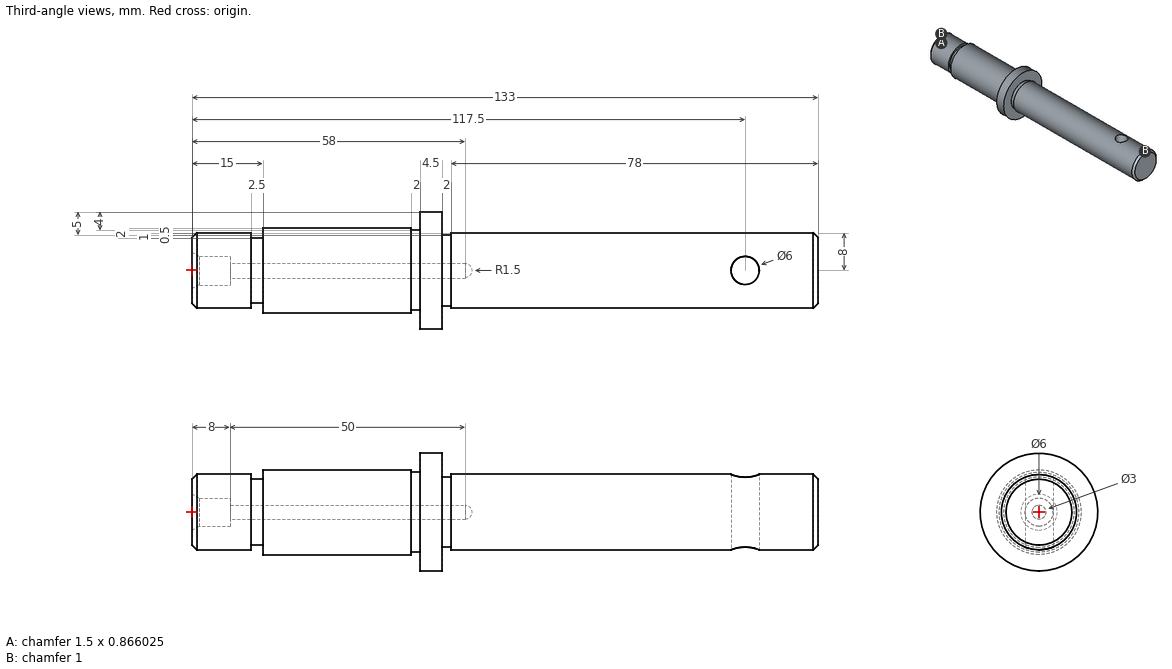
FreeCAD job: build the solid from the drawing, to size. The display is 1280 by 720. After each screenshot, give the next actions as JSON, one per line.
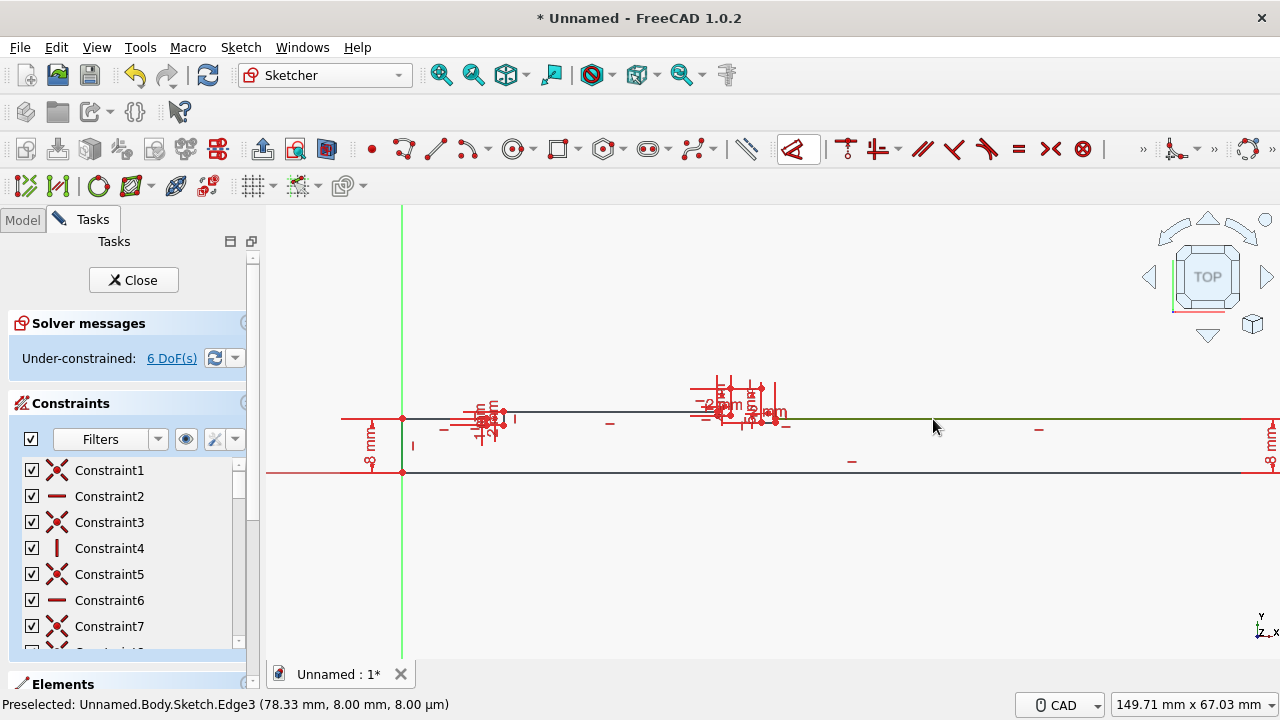
{"action": "left_click", "coordinate": [814, 150]}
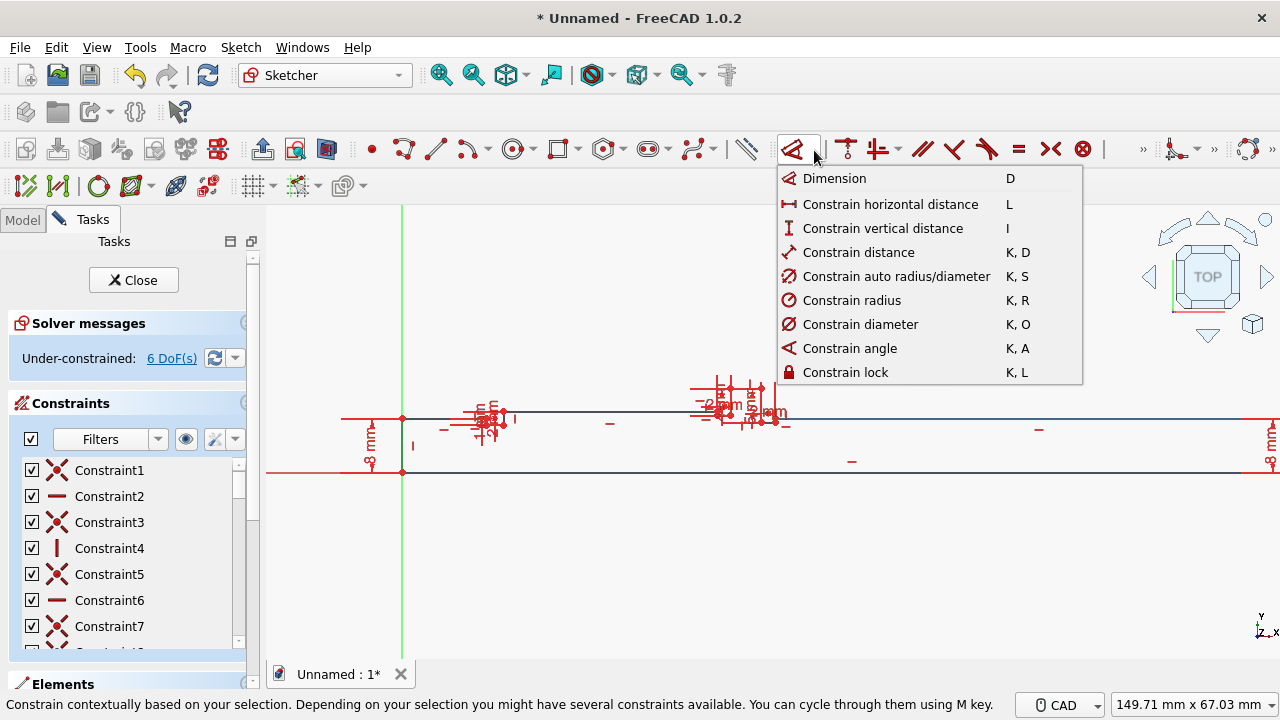
{"action": "left_click", "coordinate": [930, 204]}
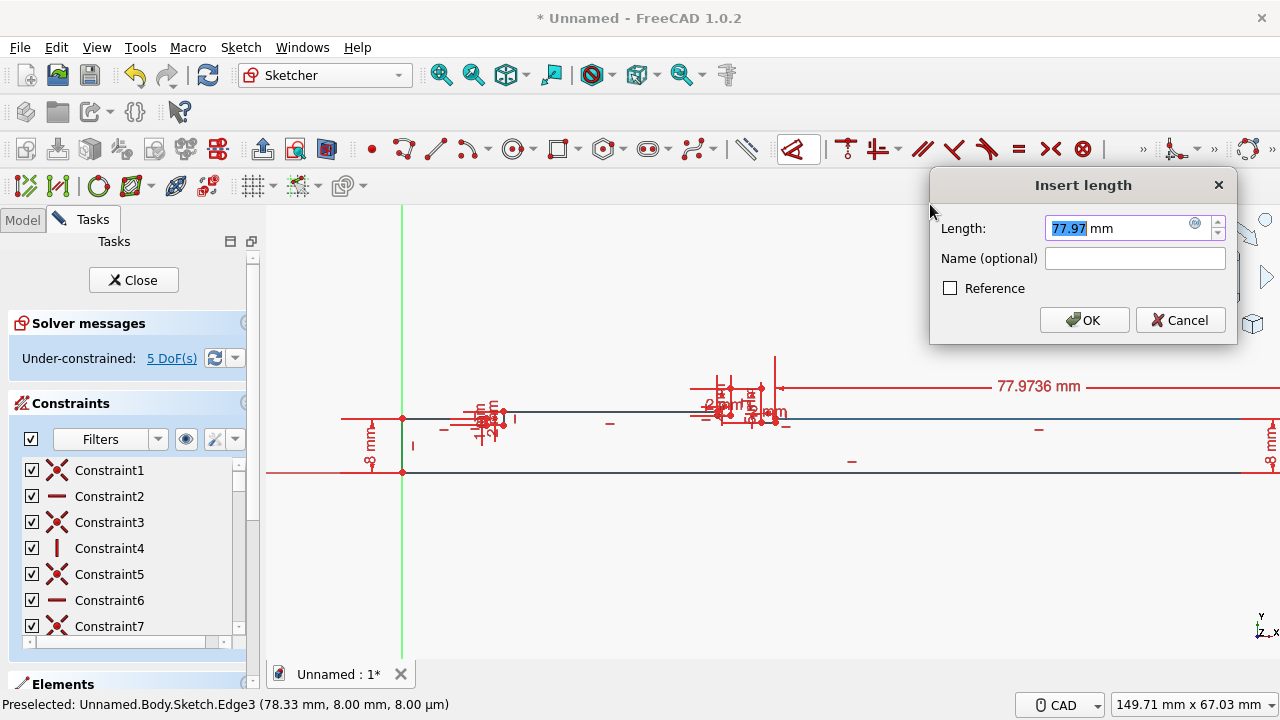
{"action": "type", "text": "78"}
{"action": "key", "text": "Return"}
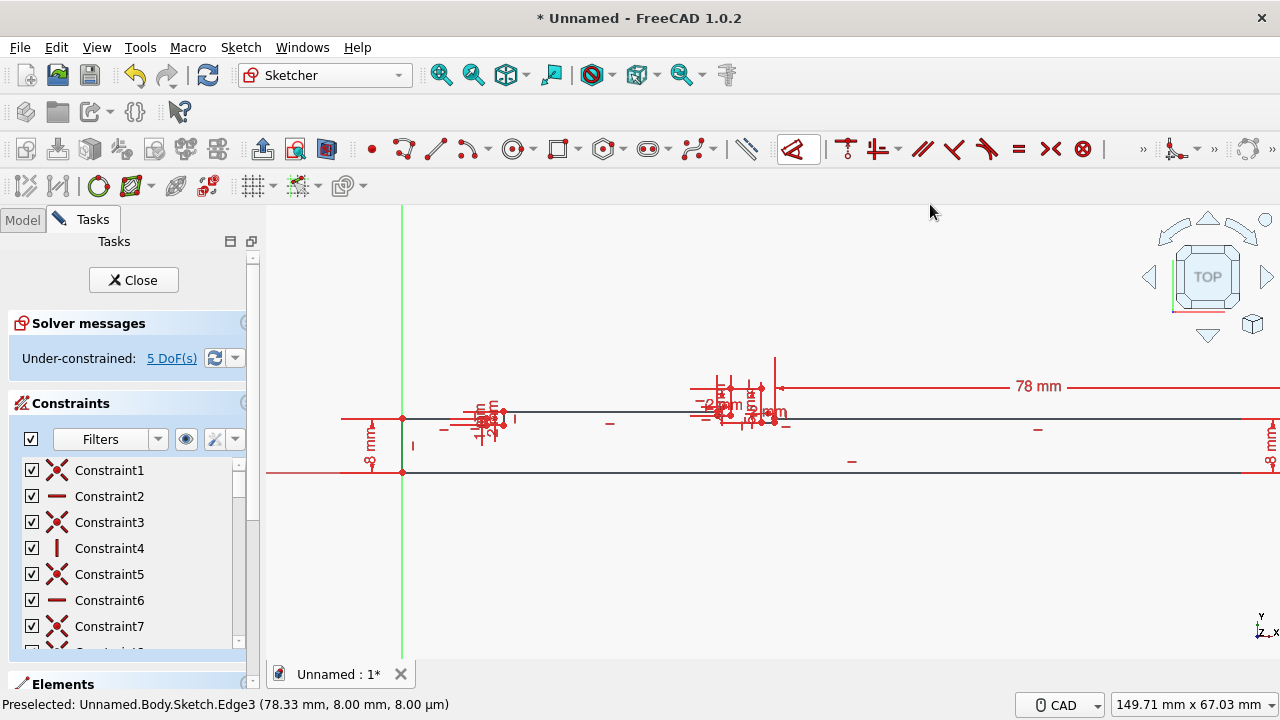
{"action": "left_click", "coordinate": [673, 473]}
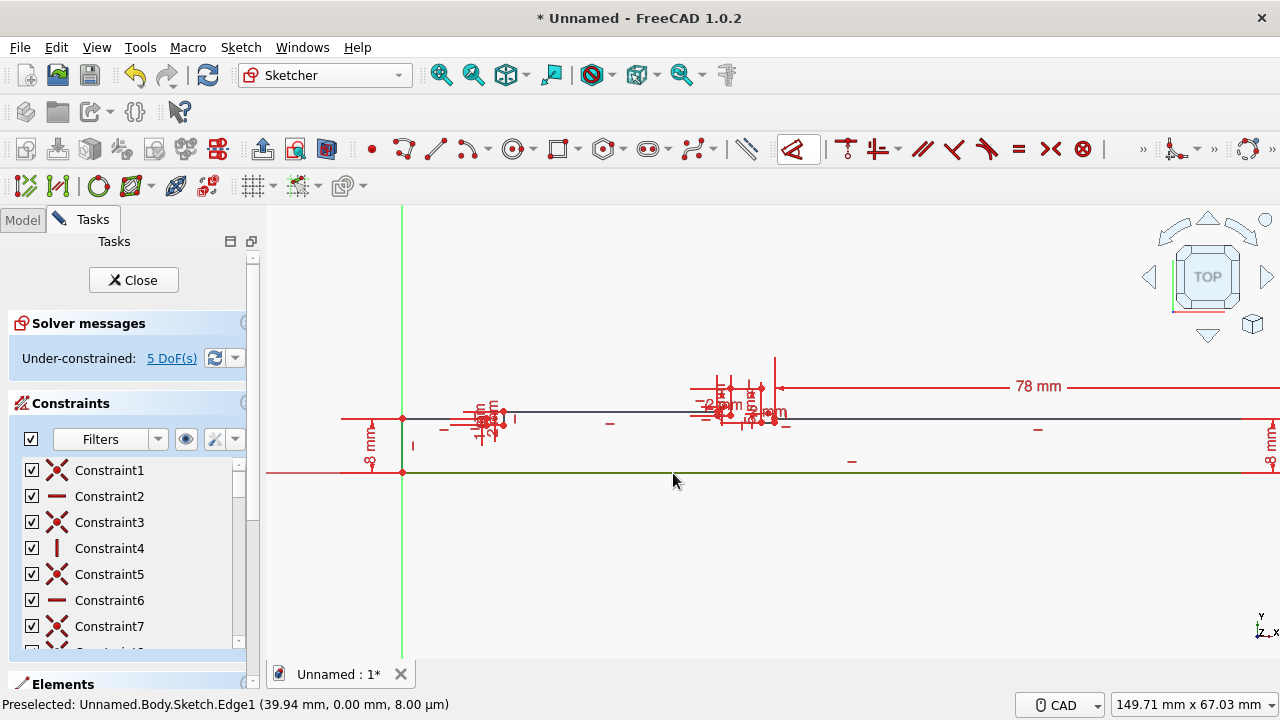
{"action": "left_click", "coordinate": [814, 150]}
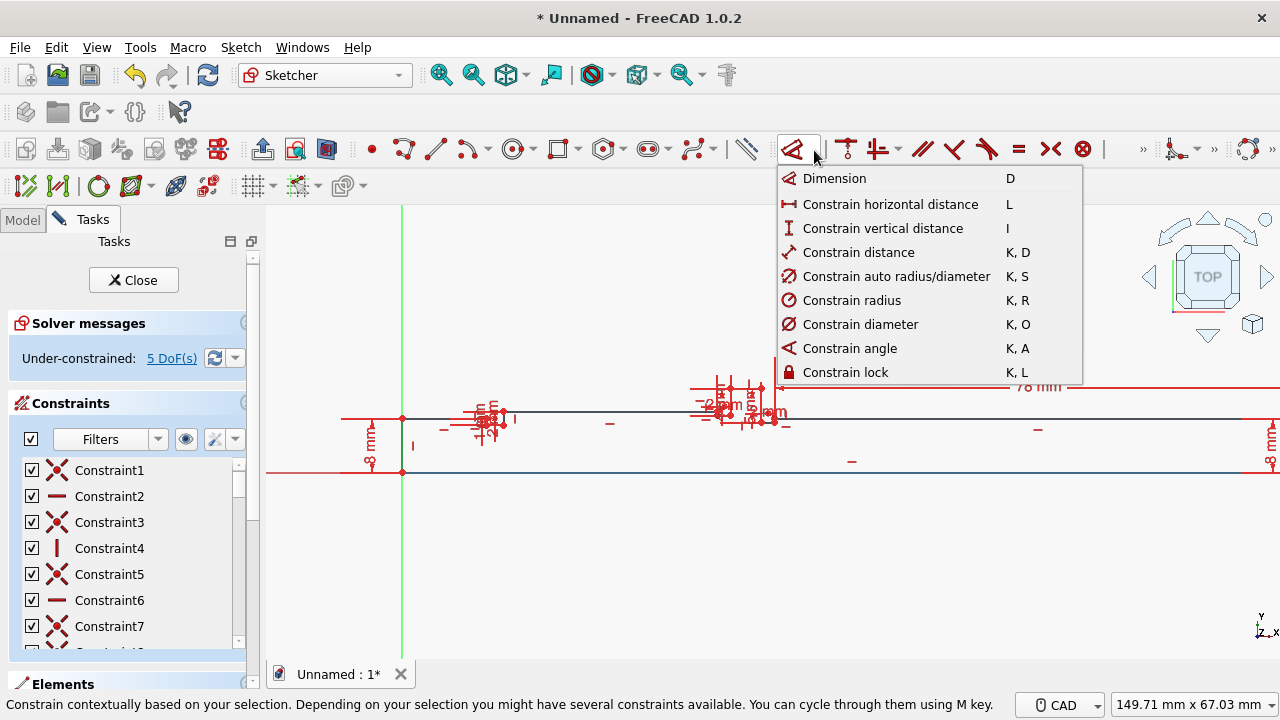
{"action": "left_click", "coordinate": [930, 204]}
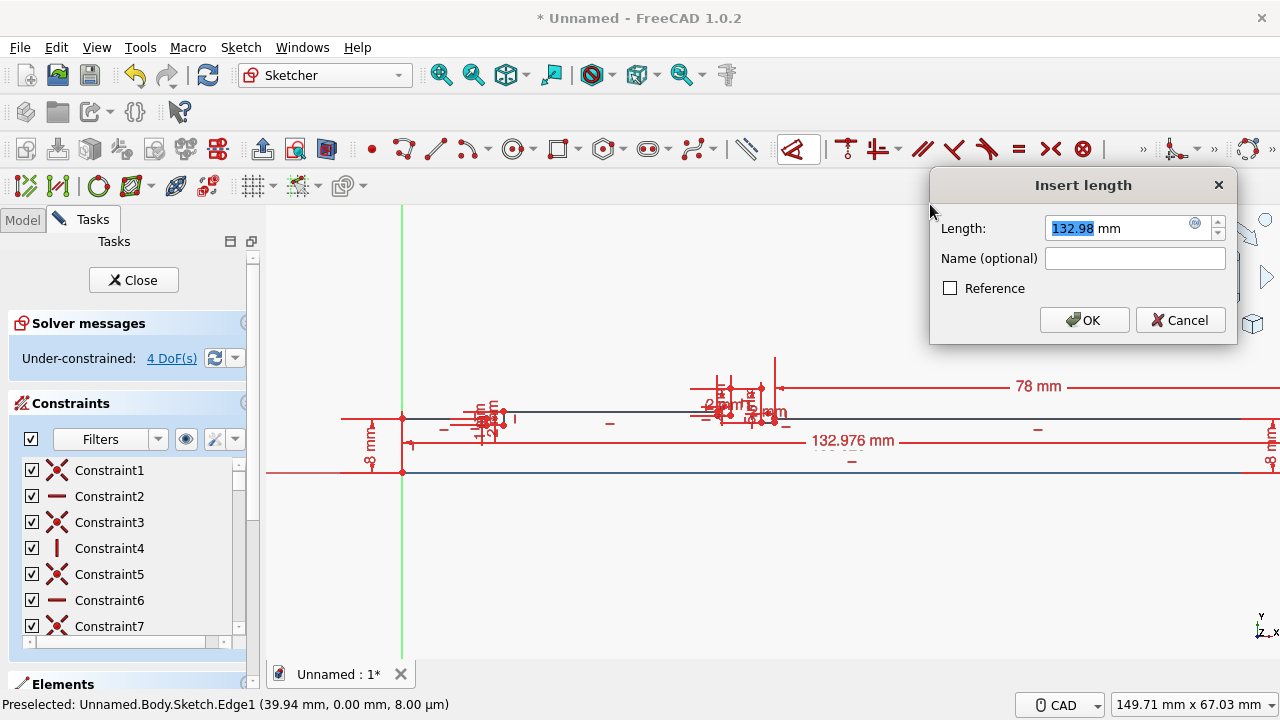
{"action": "type", "text": "133"}
{"action": "key", "text": "Return"}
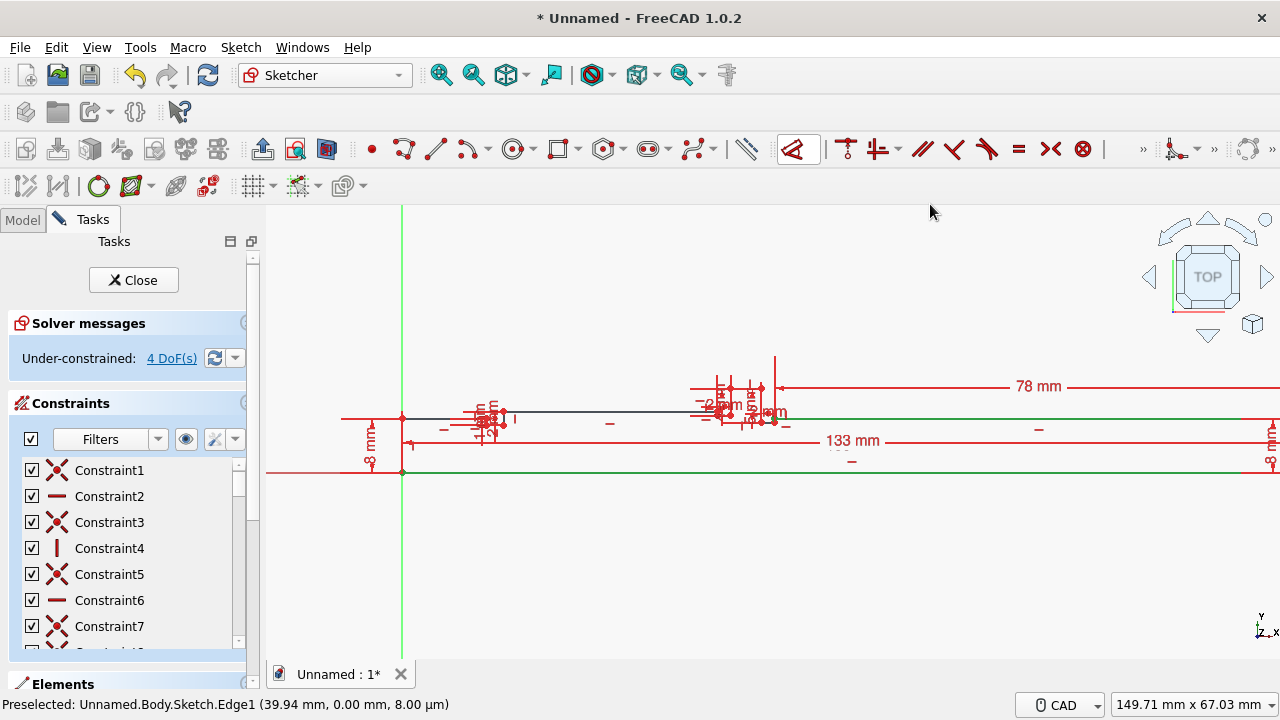
{"action": "scroll", "coordinate": [775, 421], "scroll_direction": "up", "scroll_amount": 13}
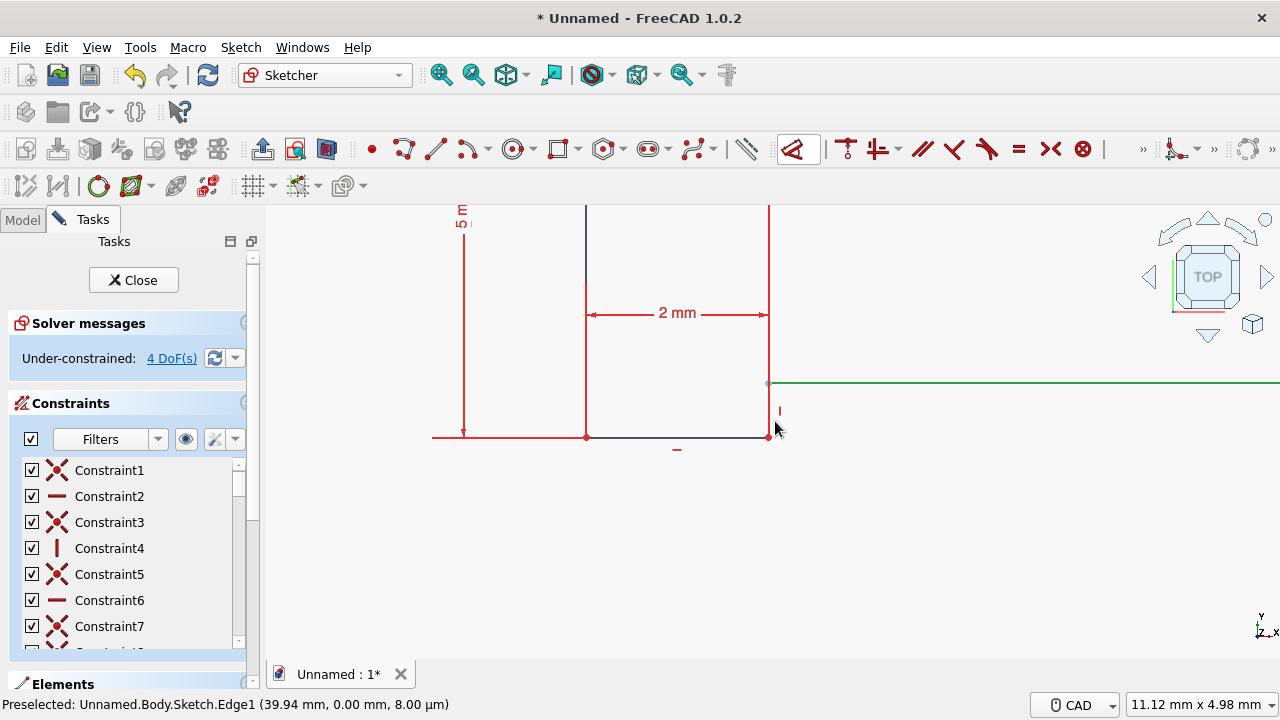
{"action": "left_click", "coordinate": [769, 411]}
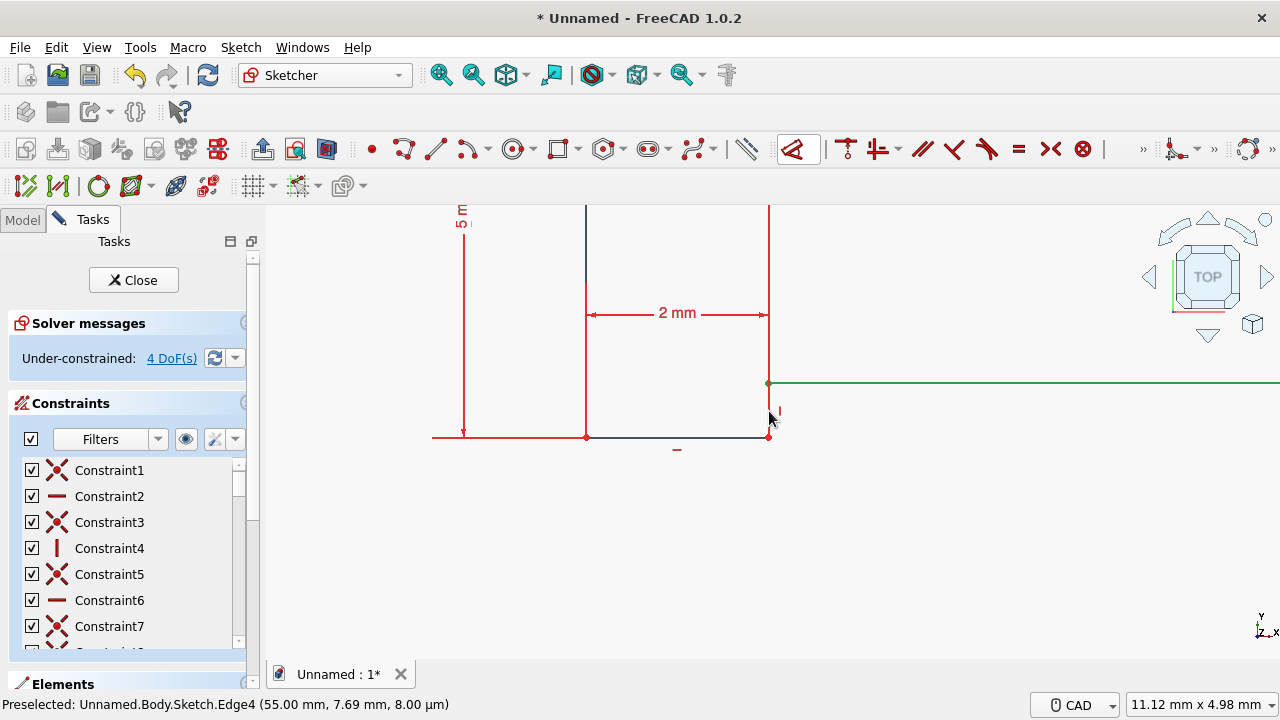
{"action": "key", "text": "i"}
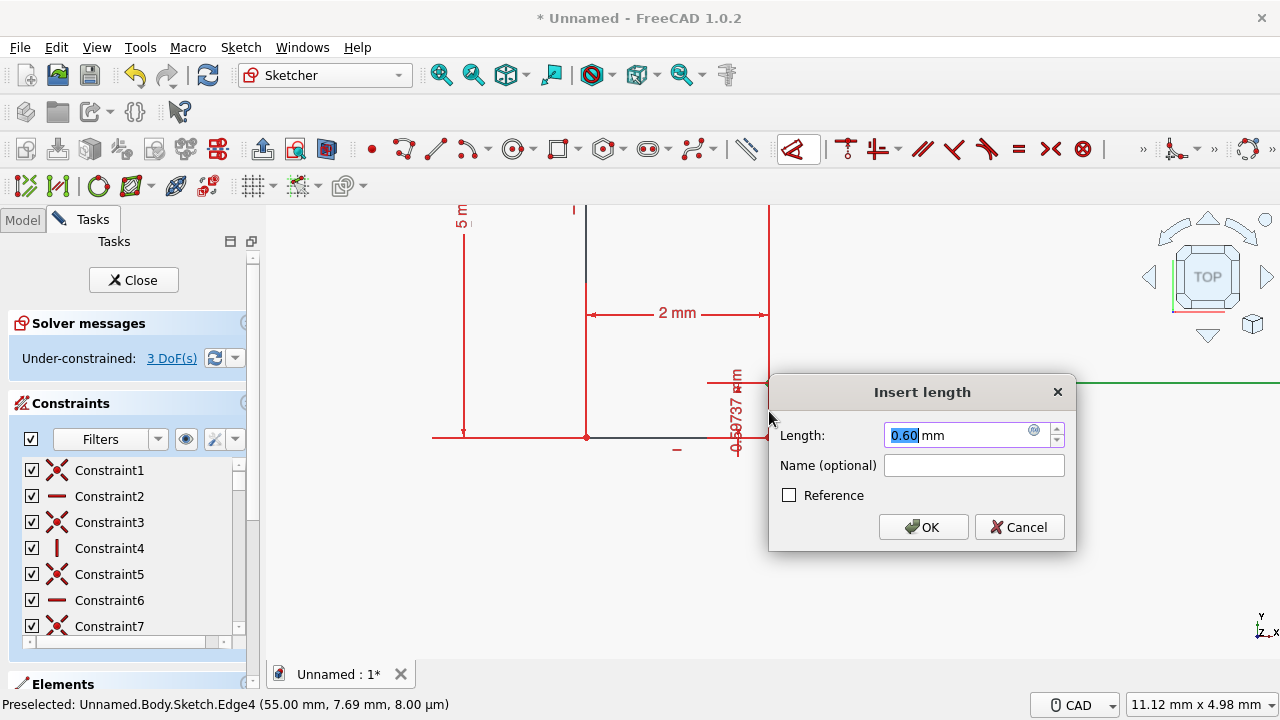
{"action": "type", "text": "0.5"}
{"action": "key", "text": "Return"}